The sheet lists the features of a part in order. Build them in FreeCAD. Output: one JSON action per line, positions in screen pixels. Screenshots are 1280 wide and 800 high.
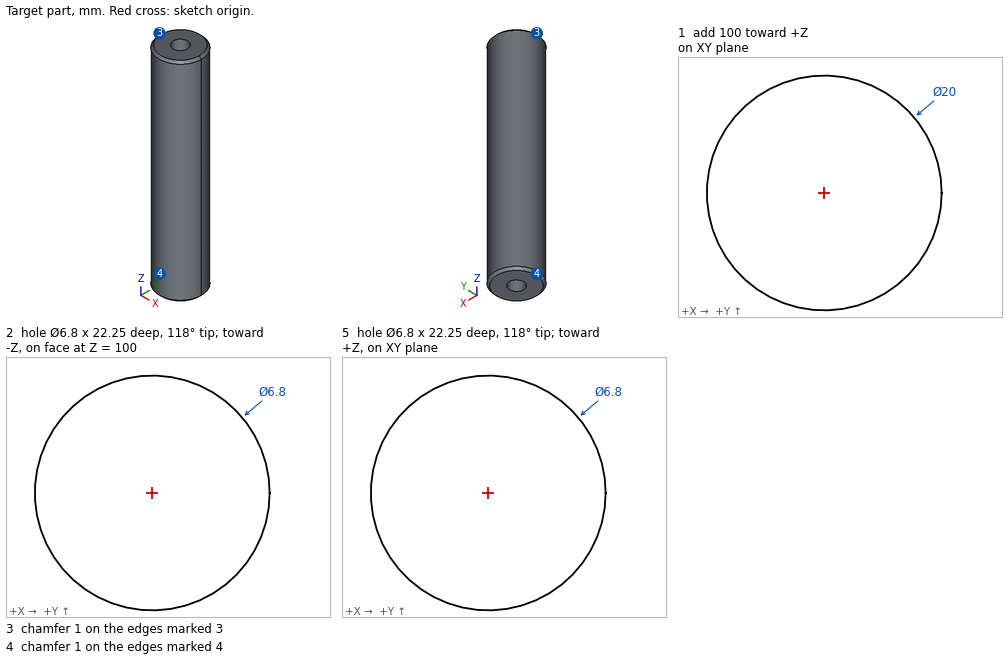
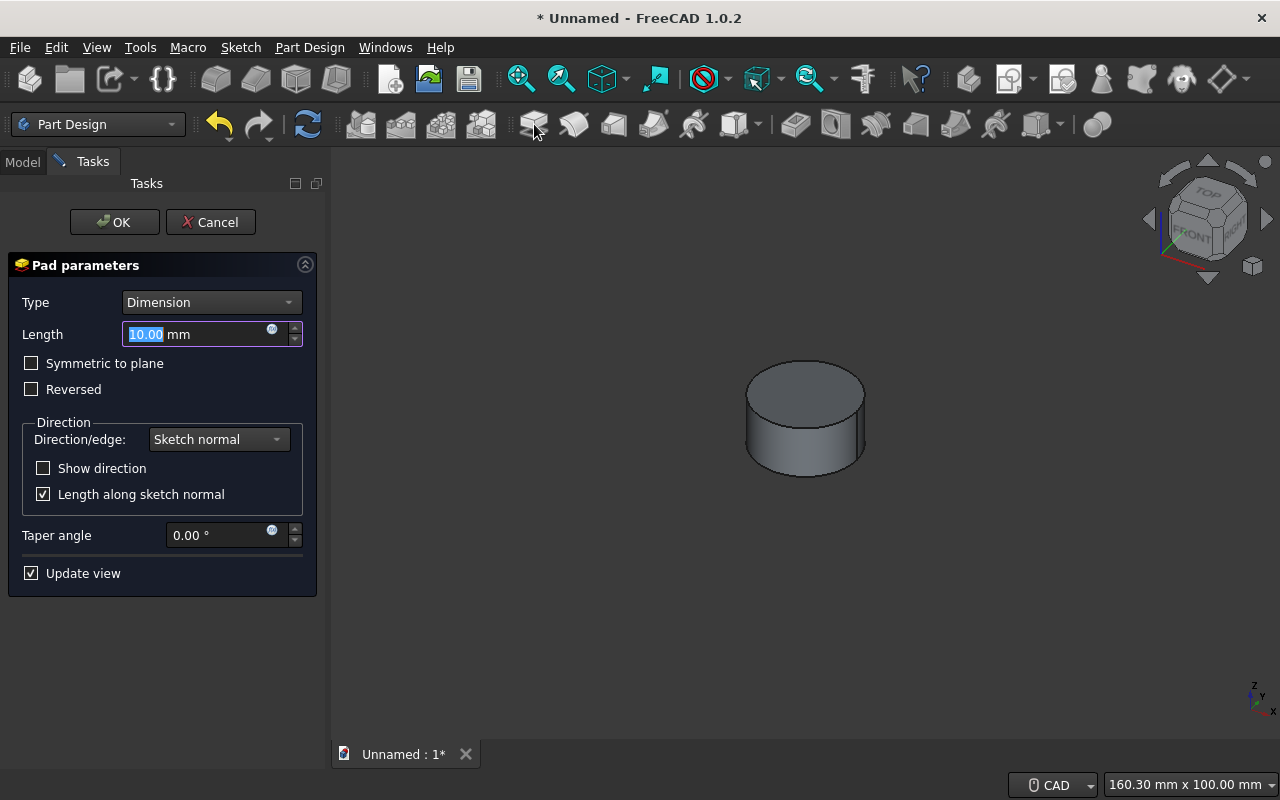
{"action": "type", "text": "100"}
{"action": "key", "text": "Tab"}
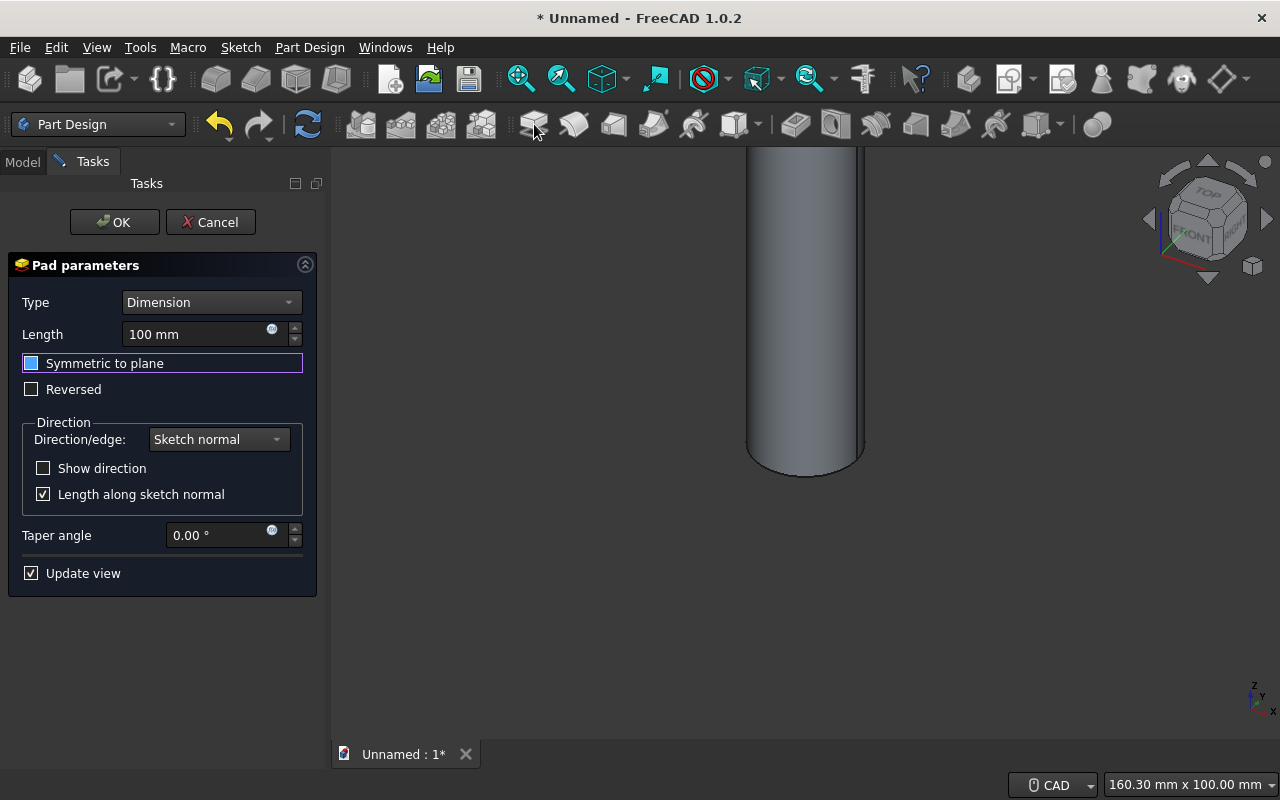
{"action": "left_click", "coordinate": [115, 222]}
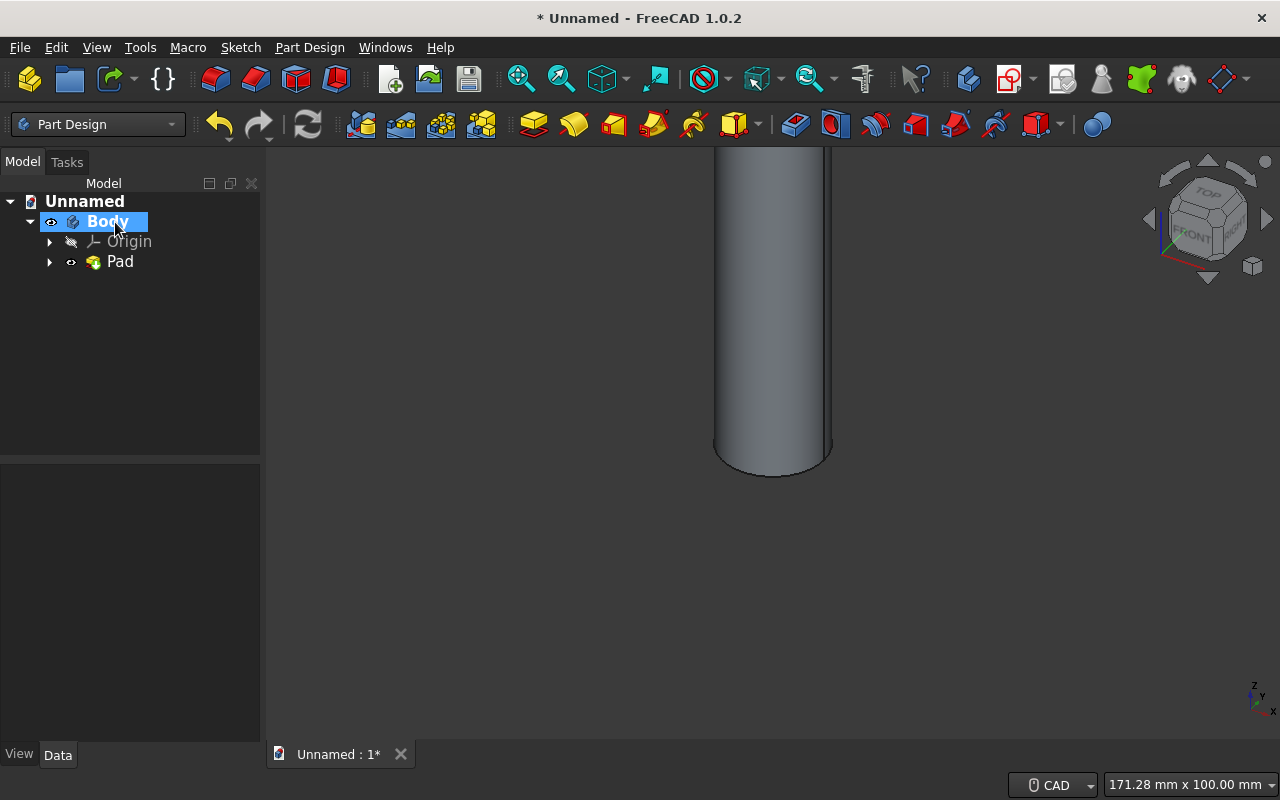
{"action": "left_click", "coordinate": [522, 80]}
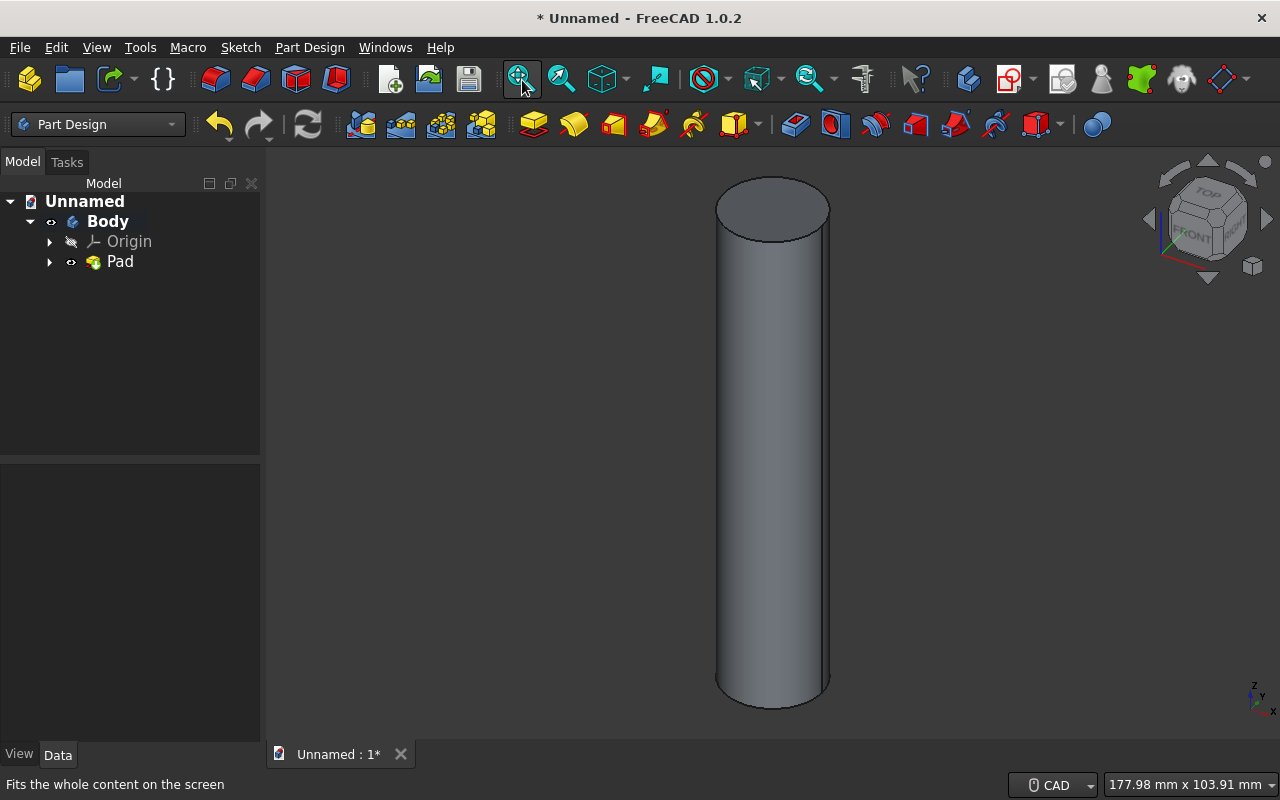
{"action": "left_click", "coordinate": [773, 209]}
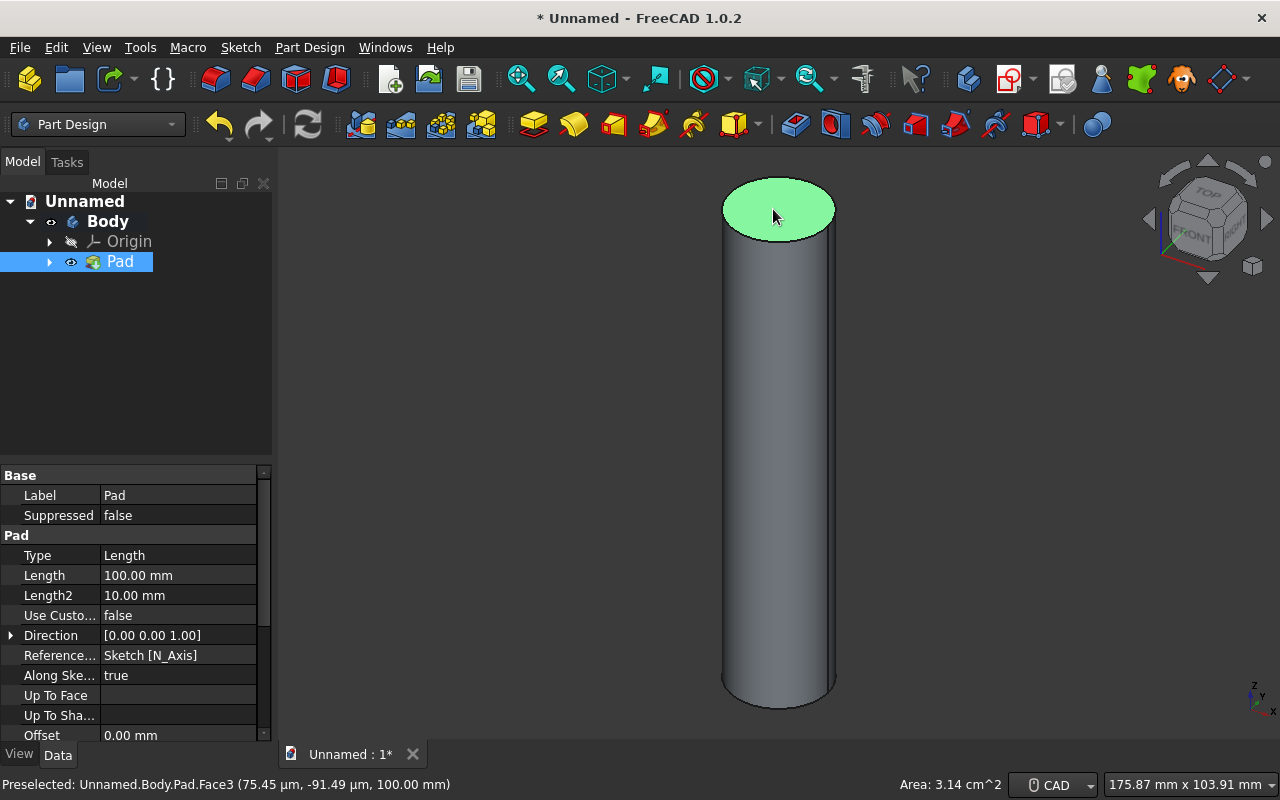
{"action": "left_click", "coordinate": [1010, 80]}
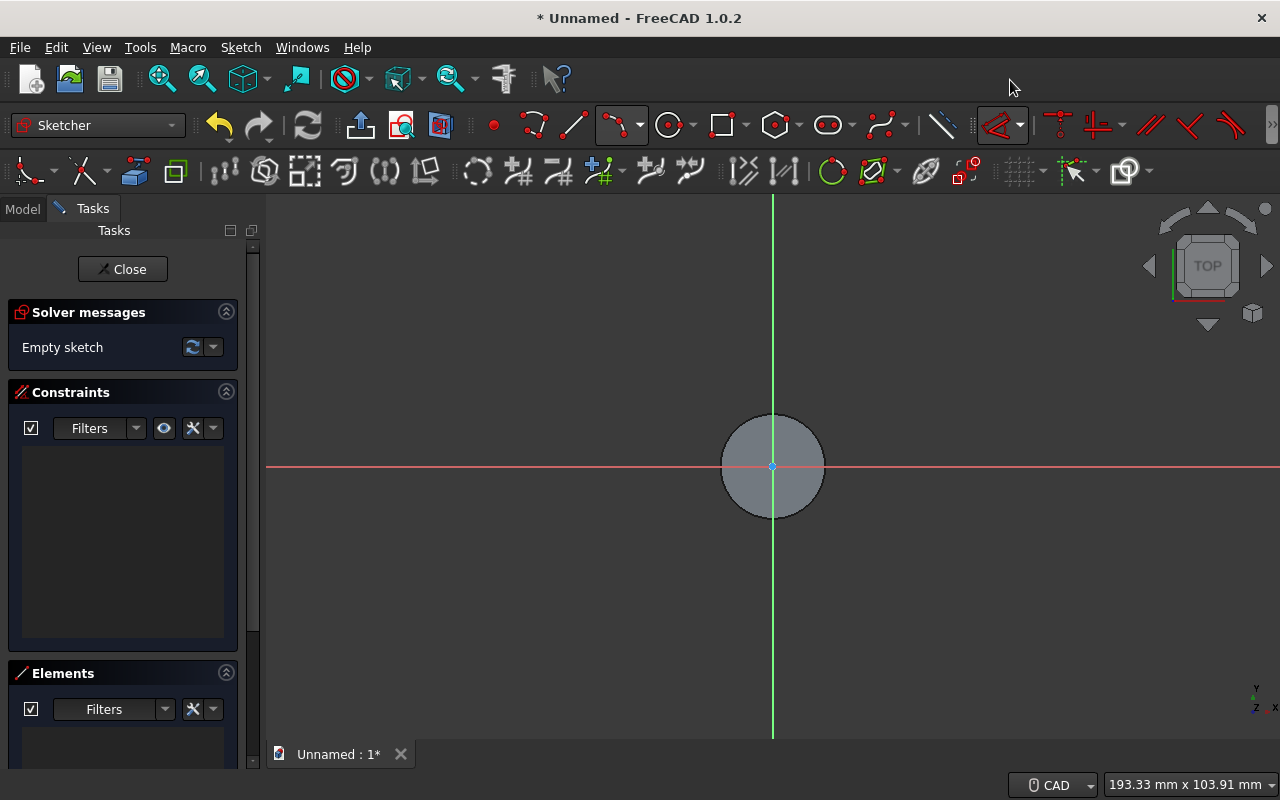
{"action": "scroll", "coordinate": [781, 466], "scroll_direction": "up", "scroll_amount": 11}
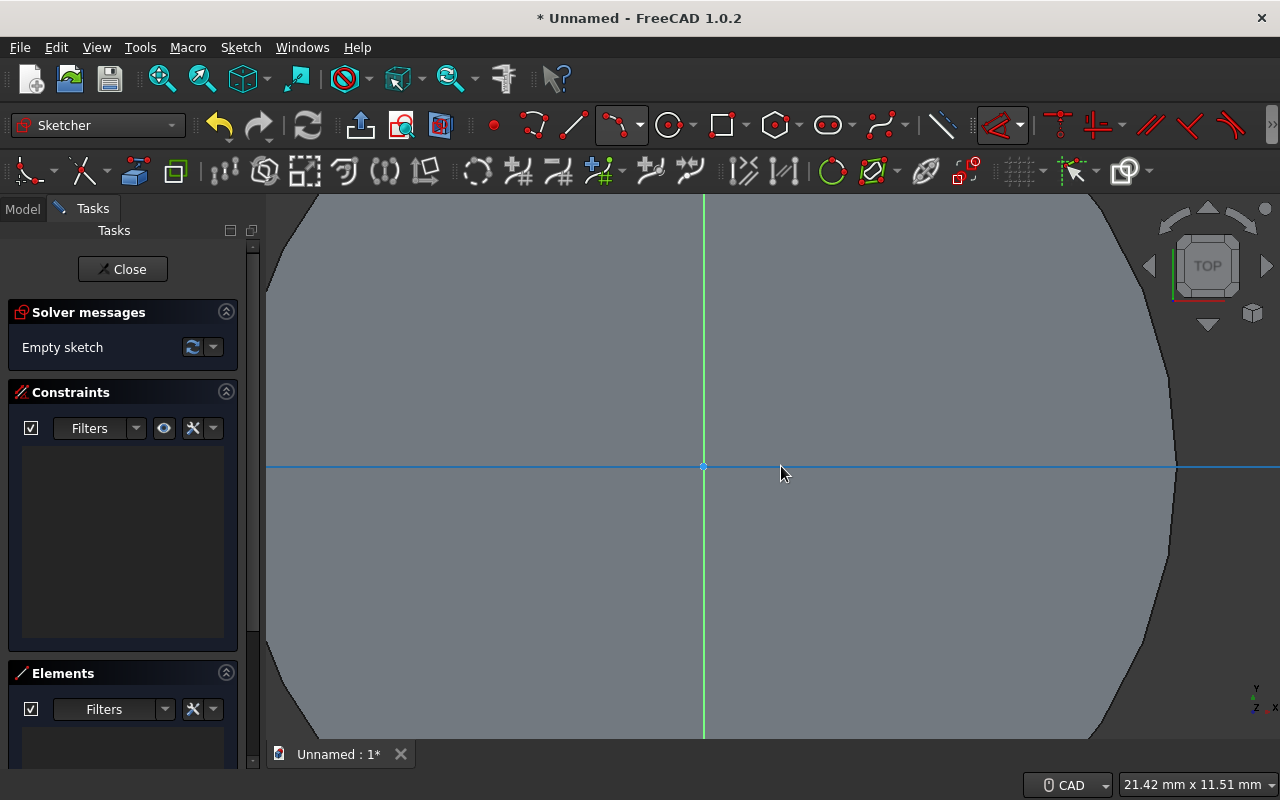
{"action": "key", "text": "g c"}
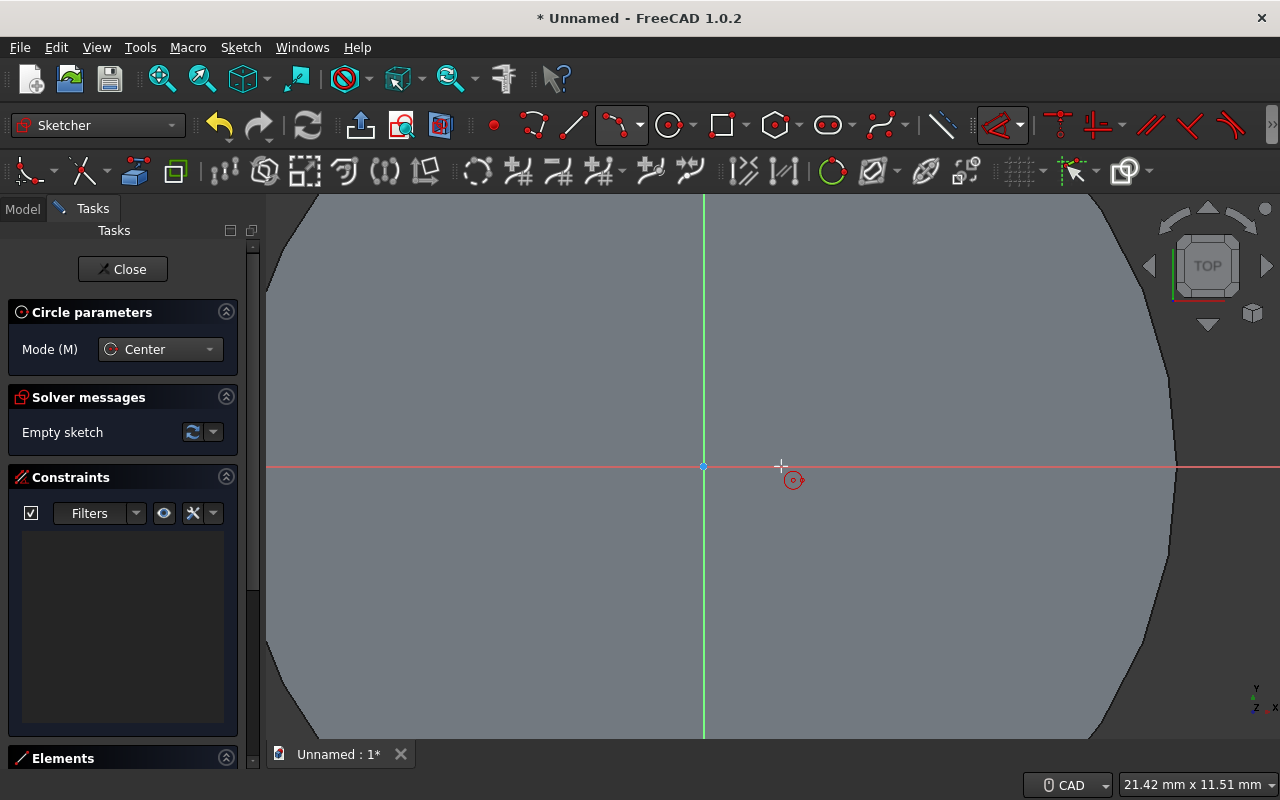
{"action": "left_click", "coordinate": [704, 466]}
{"action": "mouse_move", "coordinate": [817, 353]}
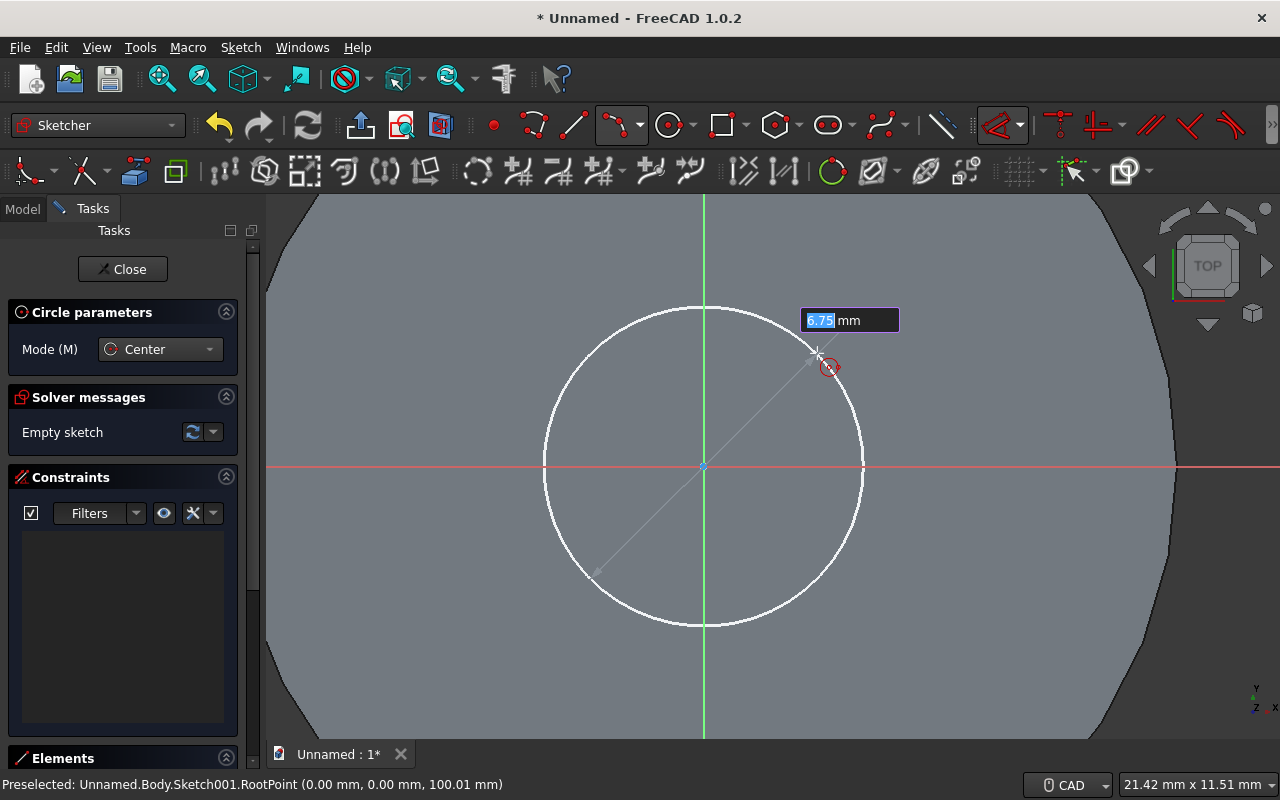
{"action": "type", "text": "6.8"}
{"action": "key", "text": "Return"}
{"action": "key", "text": "Escape"}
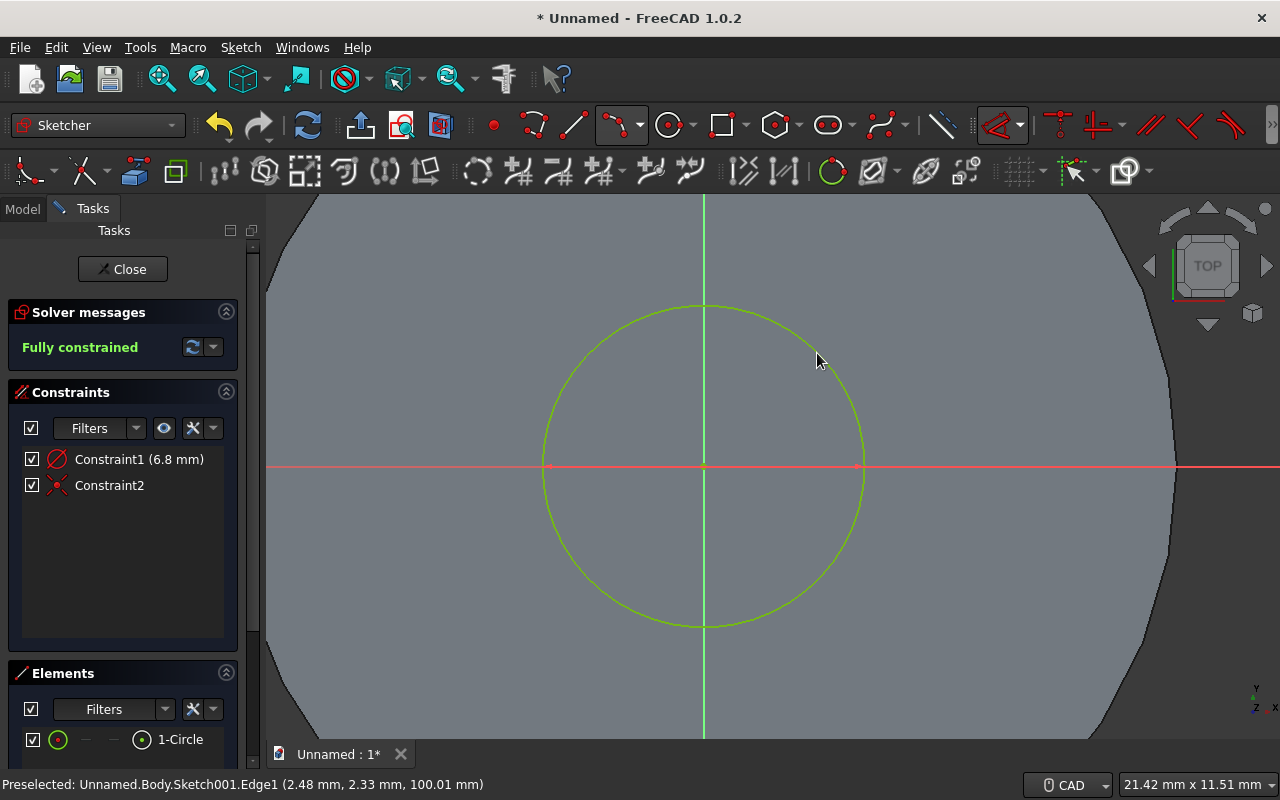
{"action": "left_click", "coordinate": [123, 269]}